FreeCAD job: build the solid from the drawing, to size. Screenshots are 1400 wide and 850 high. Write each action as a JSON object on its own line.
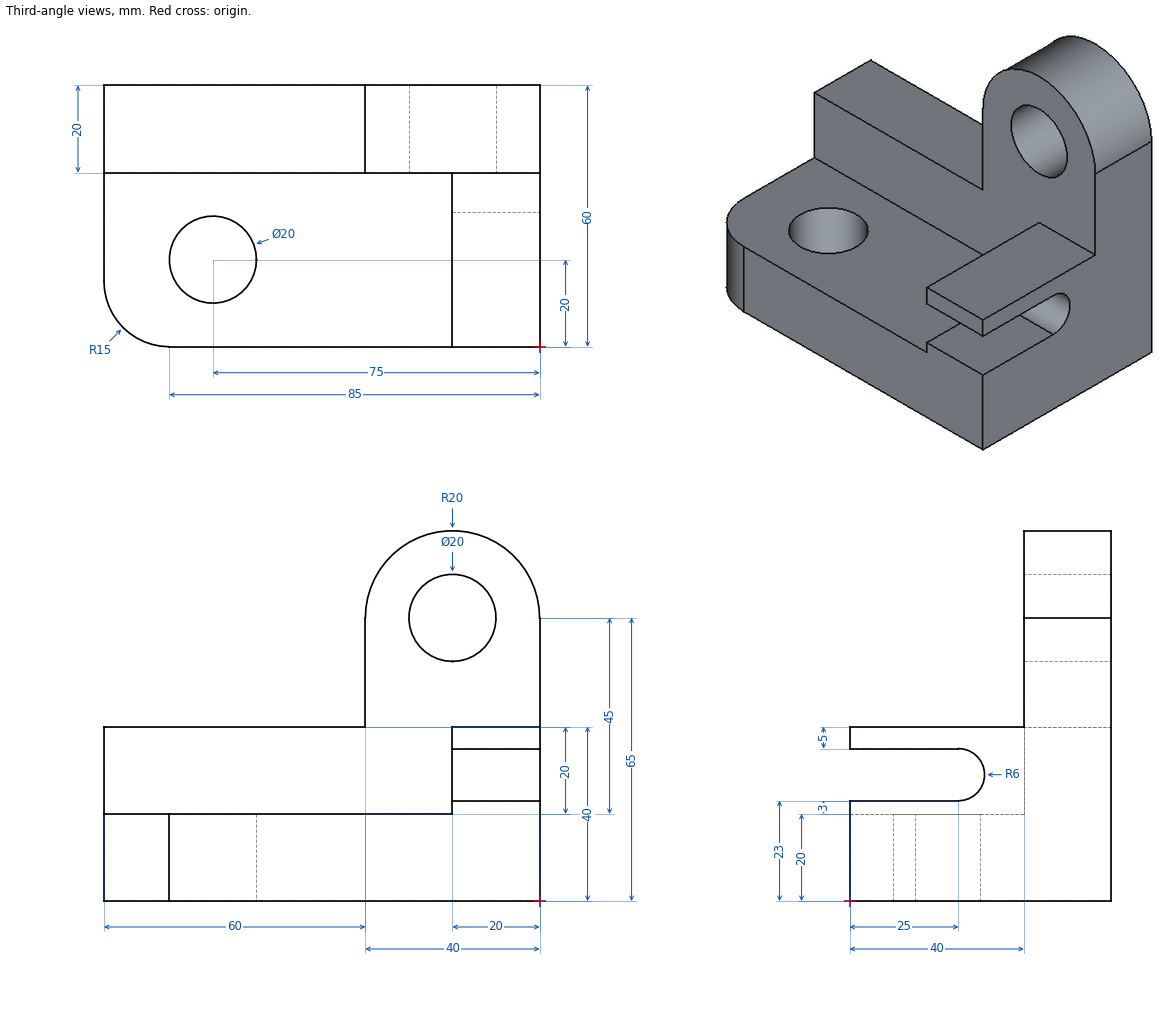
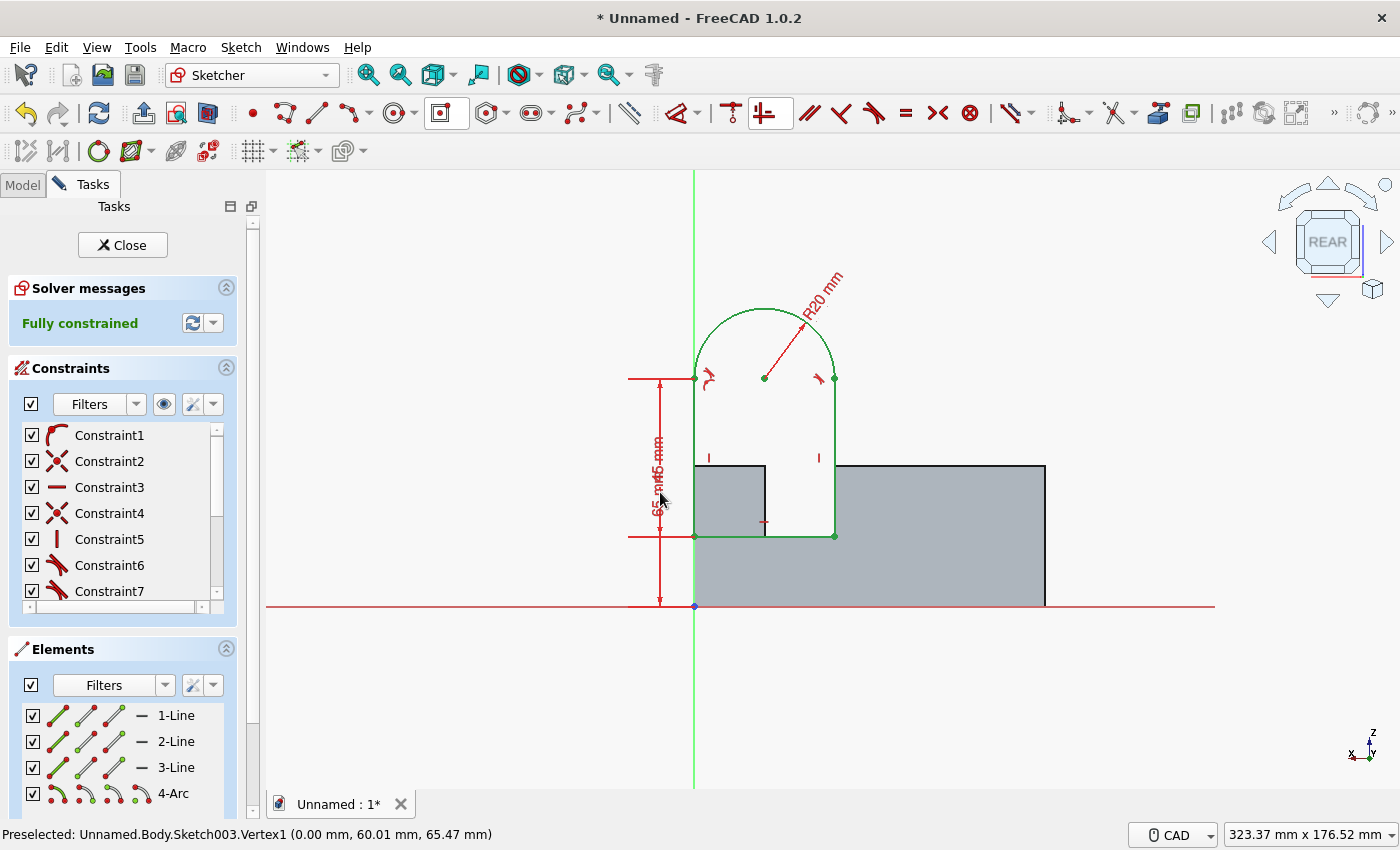
{"action": "left_click", "coordinate": [123, 245]}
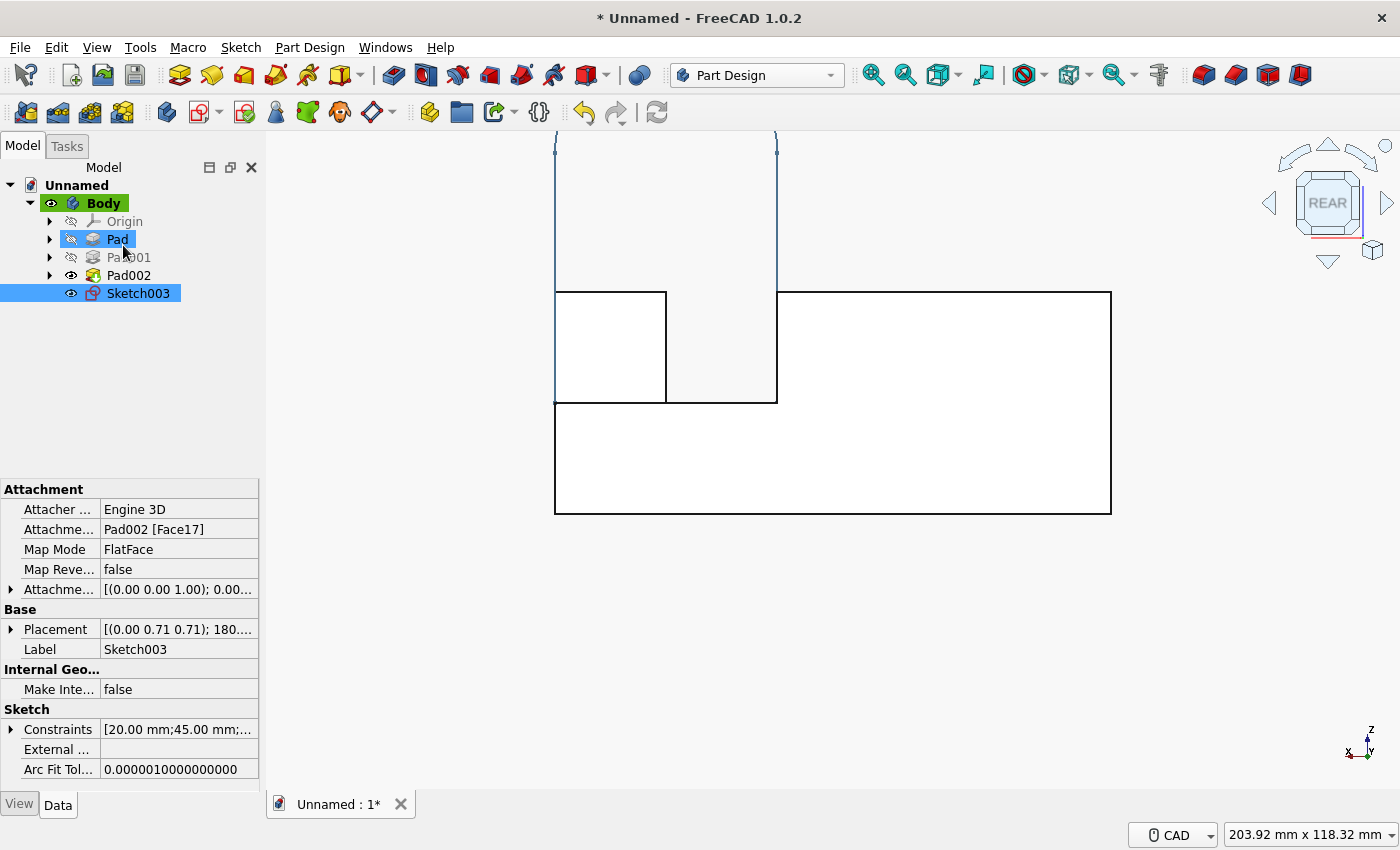
{"action": "left_click", "coordinate": [180, 76]}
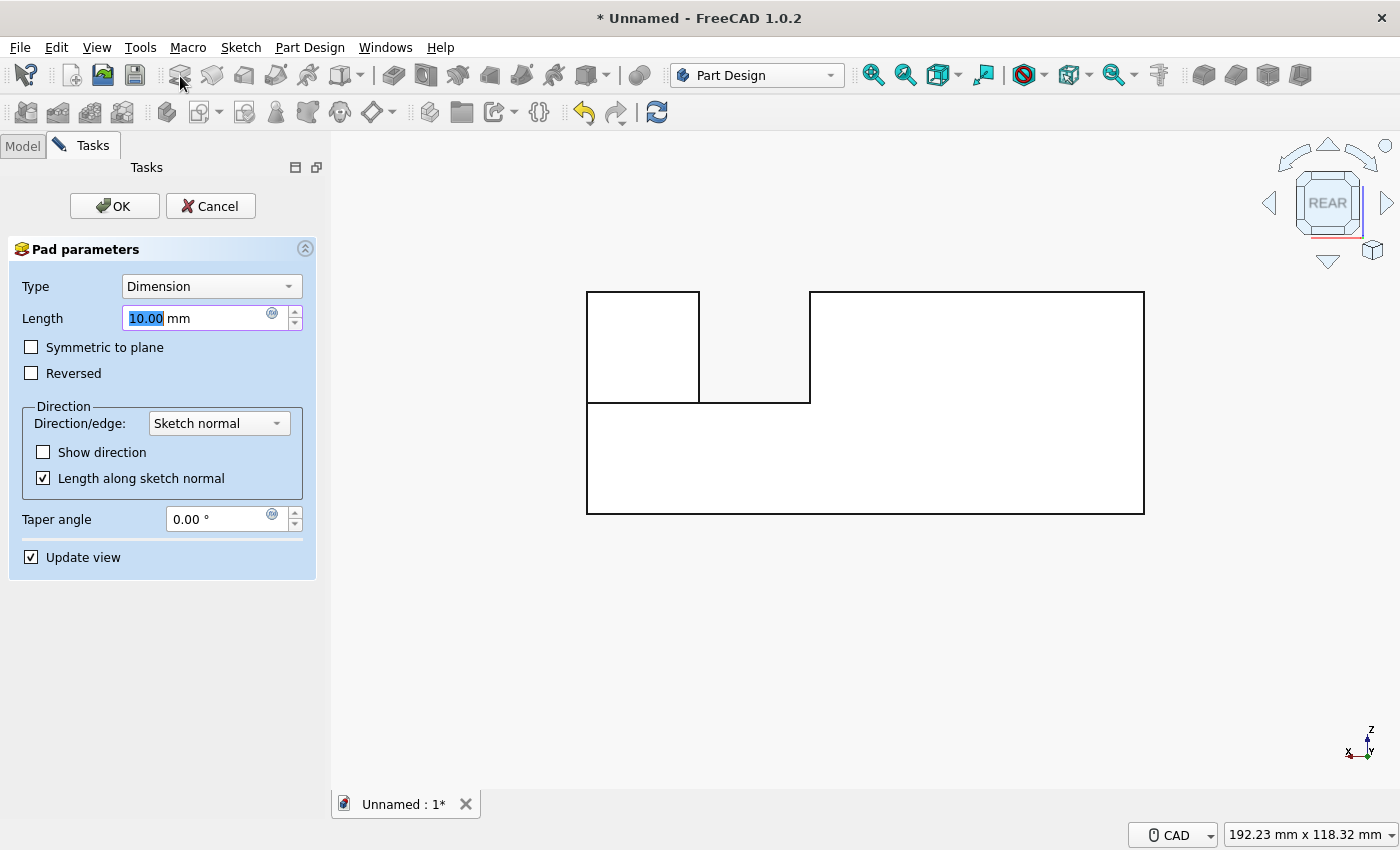
{"action": "type", "text": "20"}
{"action": "key", "text": "Tab"}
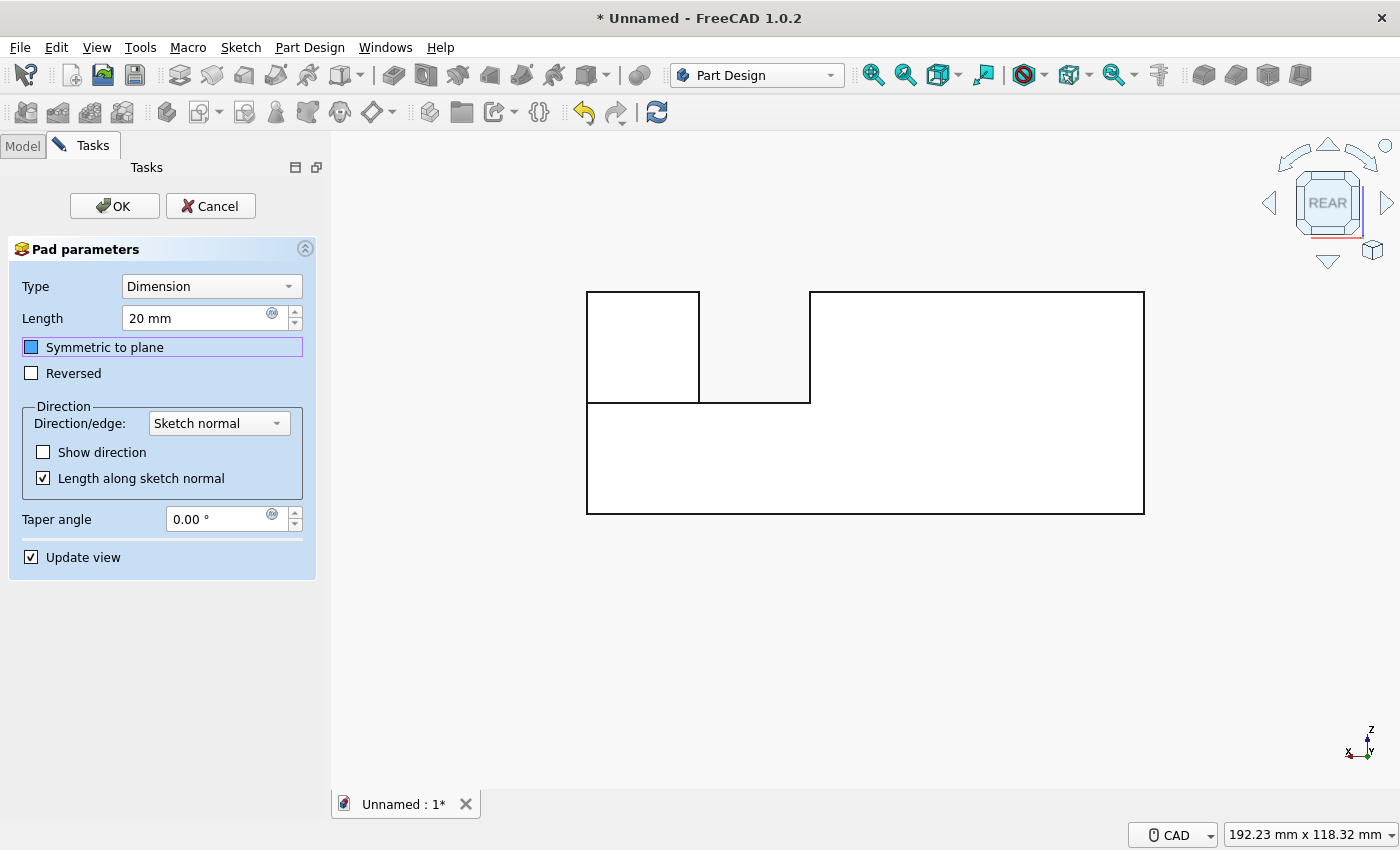
{"action": "left_click", "coordinate": [30, 373]}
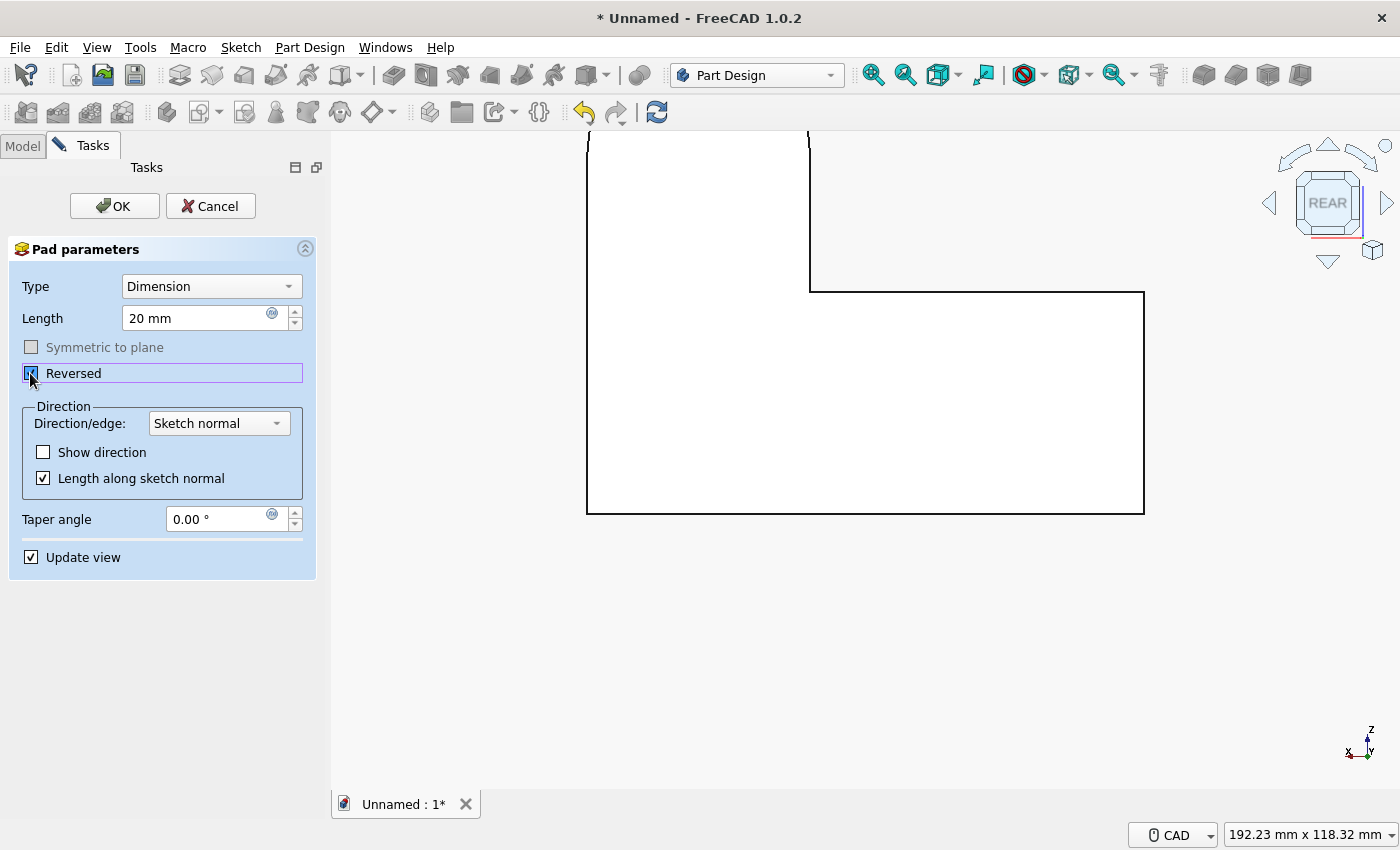
{"action": "left_click", "coordinate": [115, 206]}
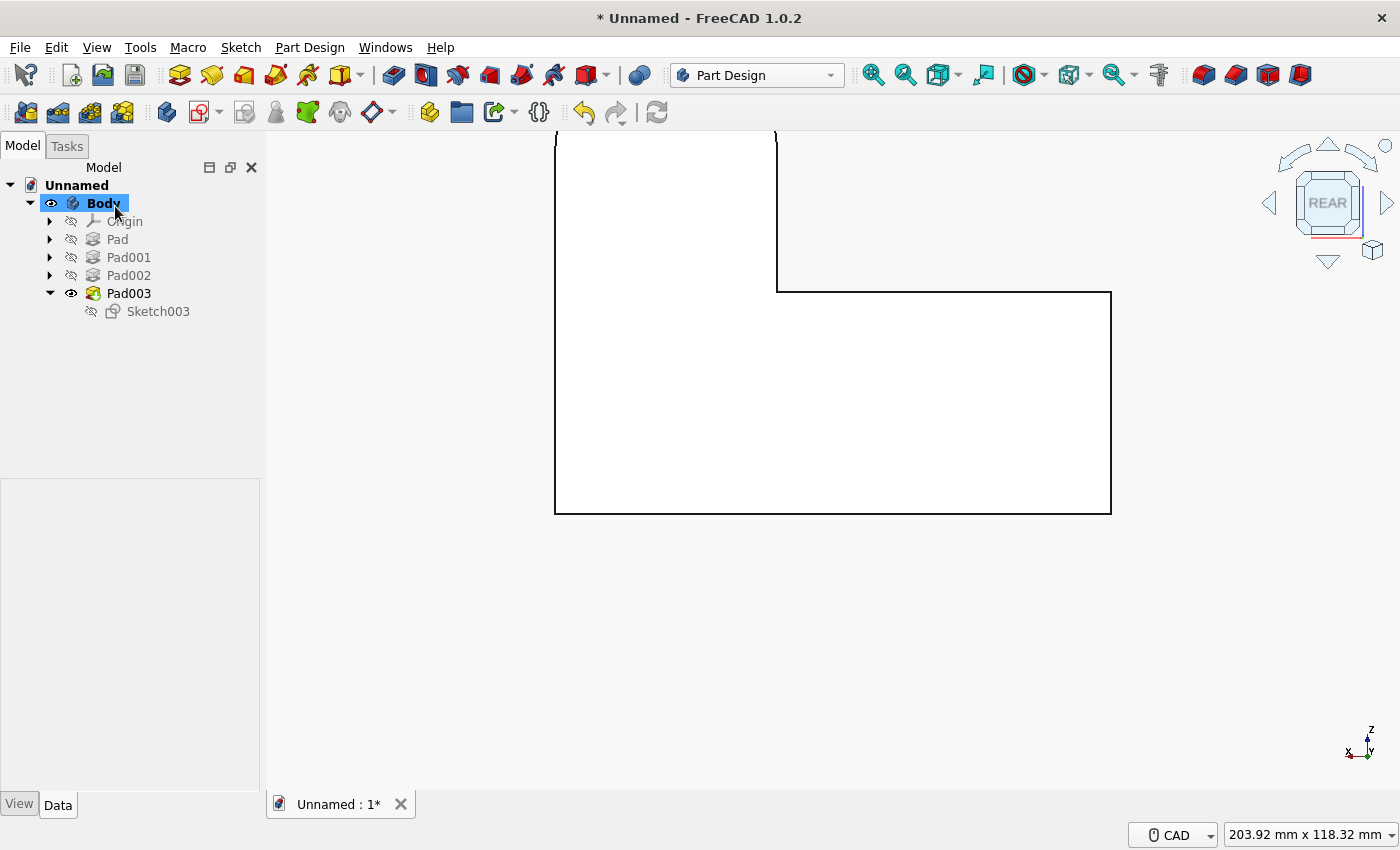
{"action": "left_click", "coordinate": [874, 76]}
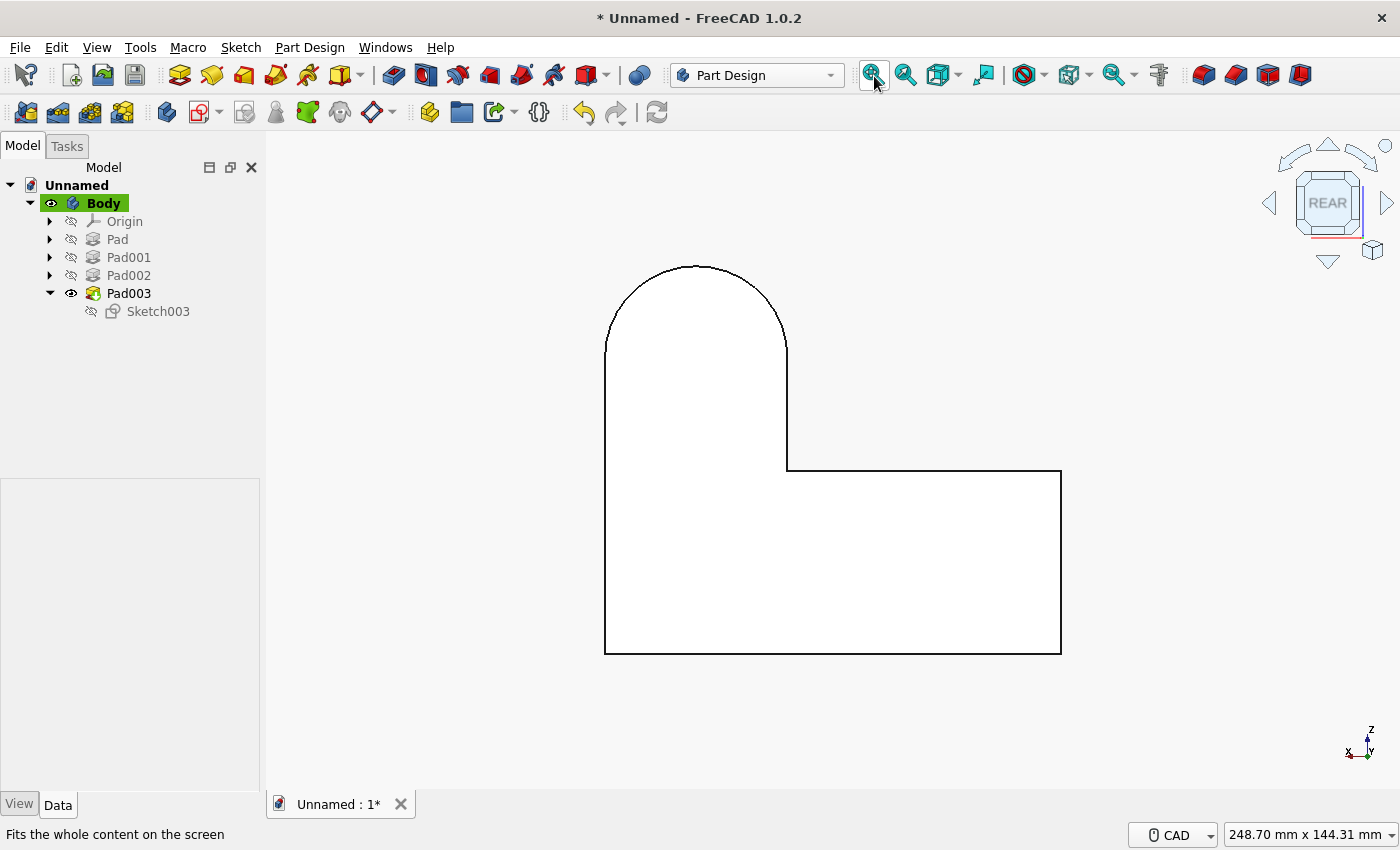
{"action": "key", "text": "0"}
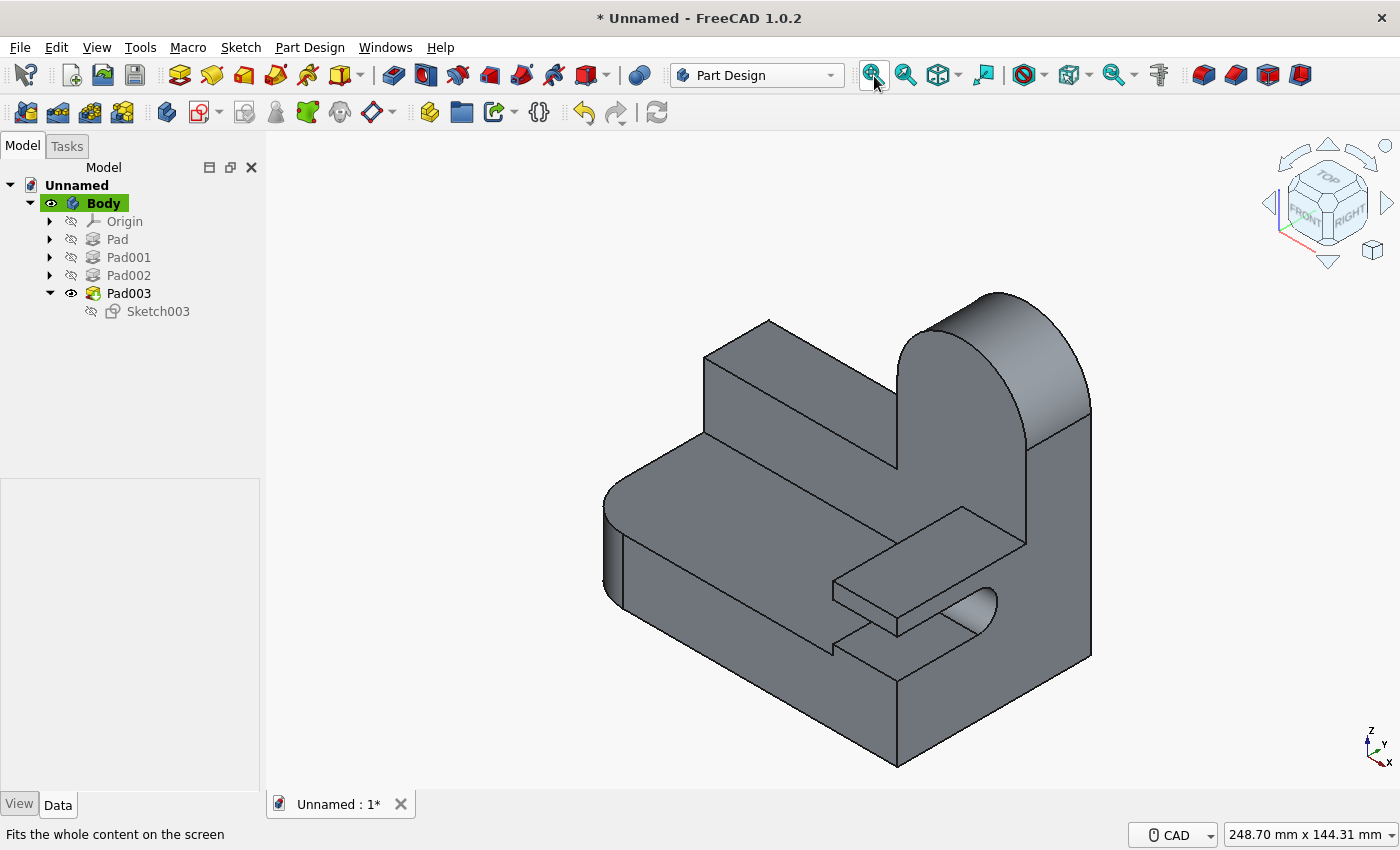
{"action": "left_click", "coordinate": [957, 422]}